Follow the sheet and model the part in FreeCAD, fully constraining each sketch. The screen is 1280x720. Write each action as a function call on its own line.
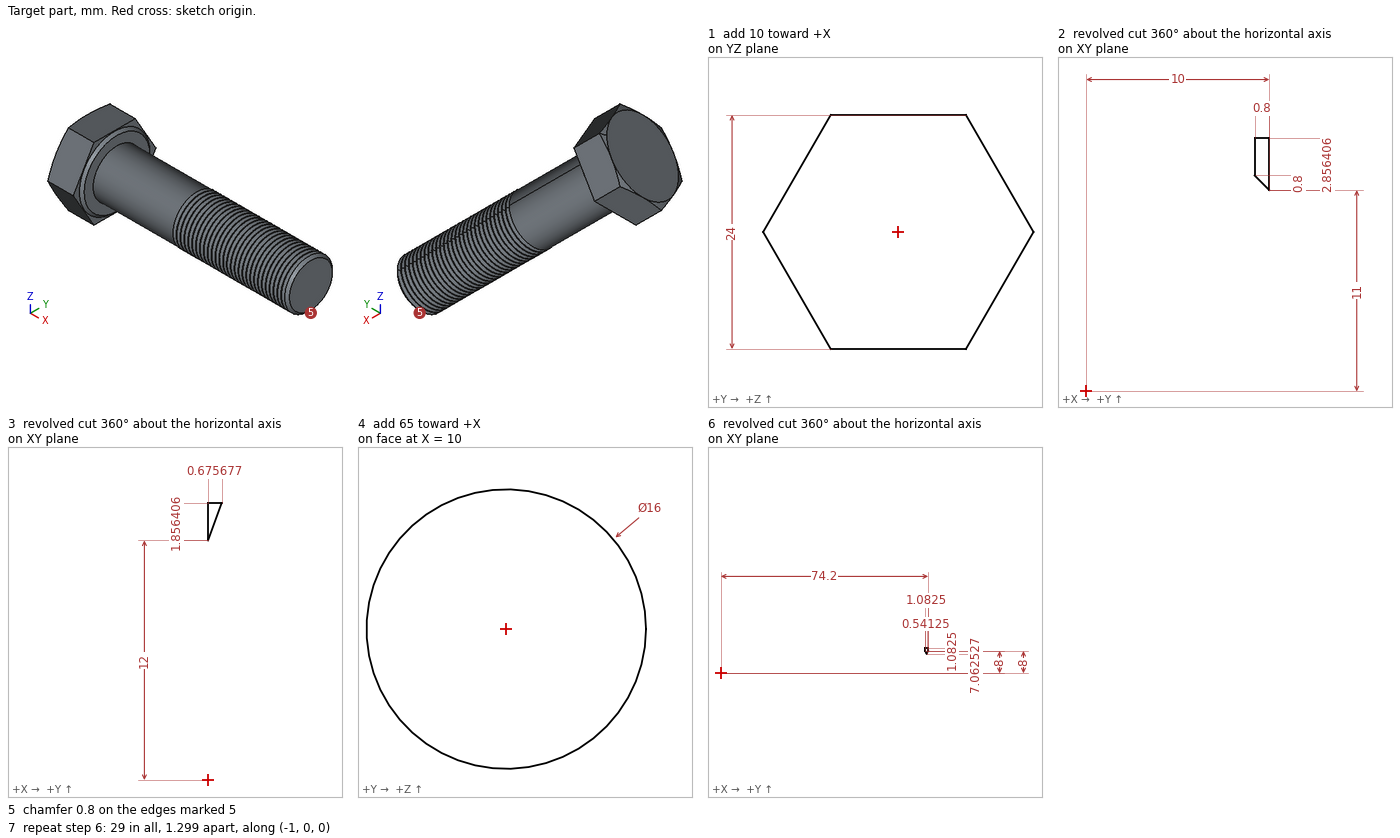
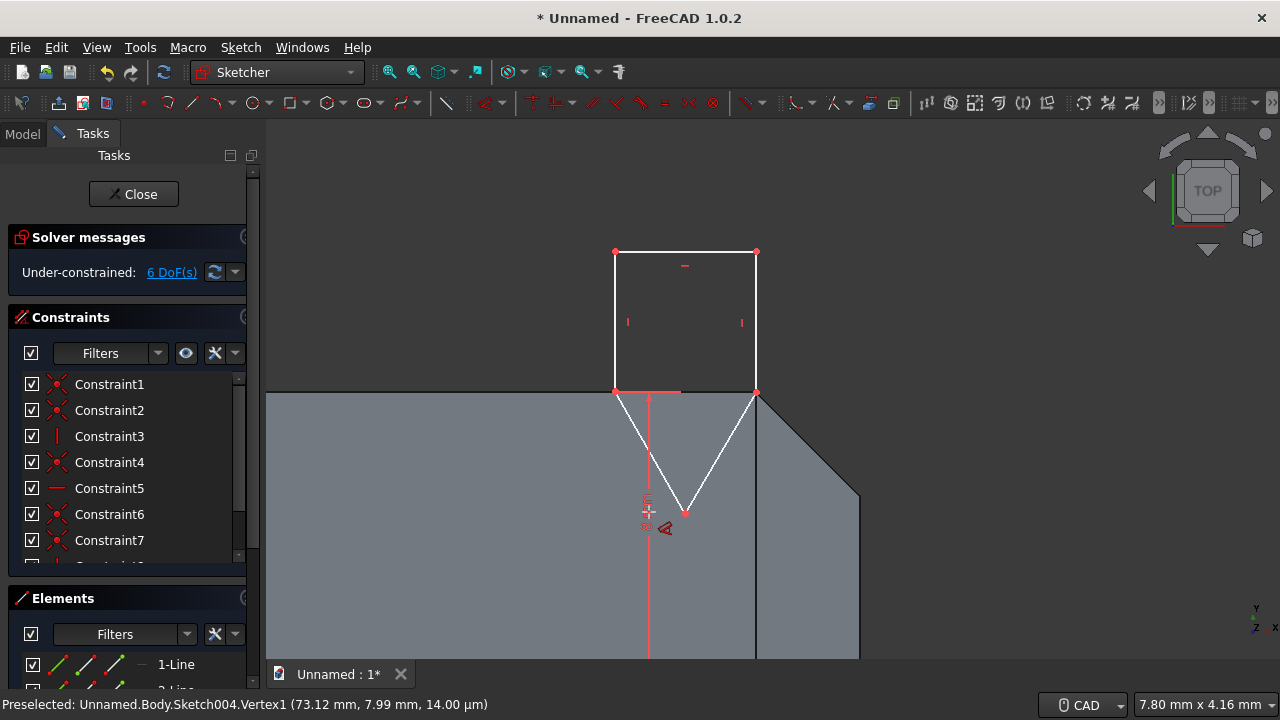
click(756, 393)
click(790, 512)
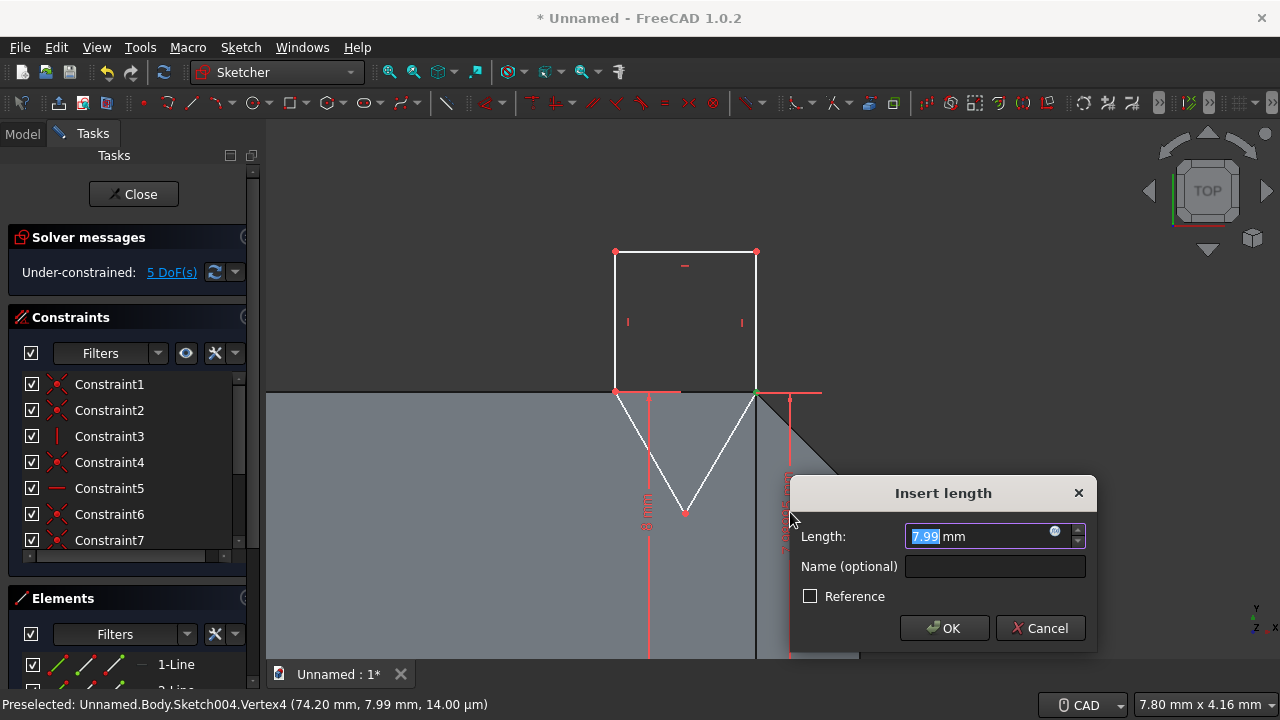
text(8)
key(Return)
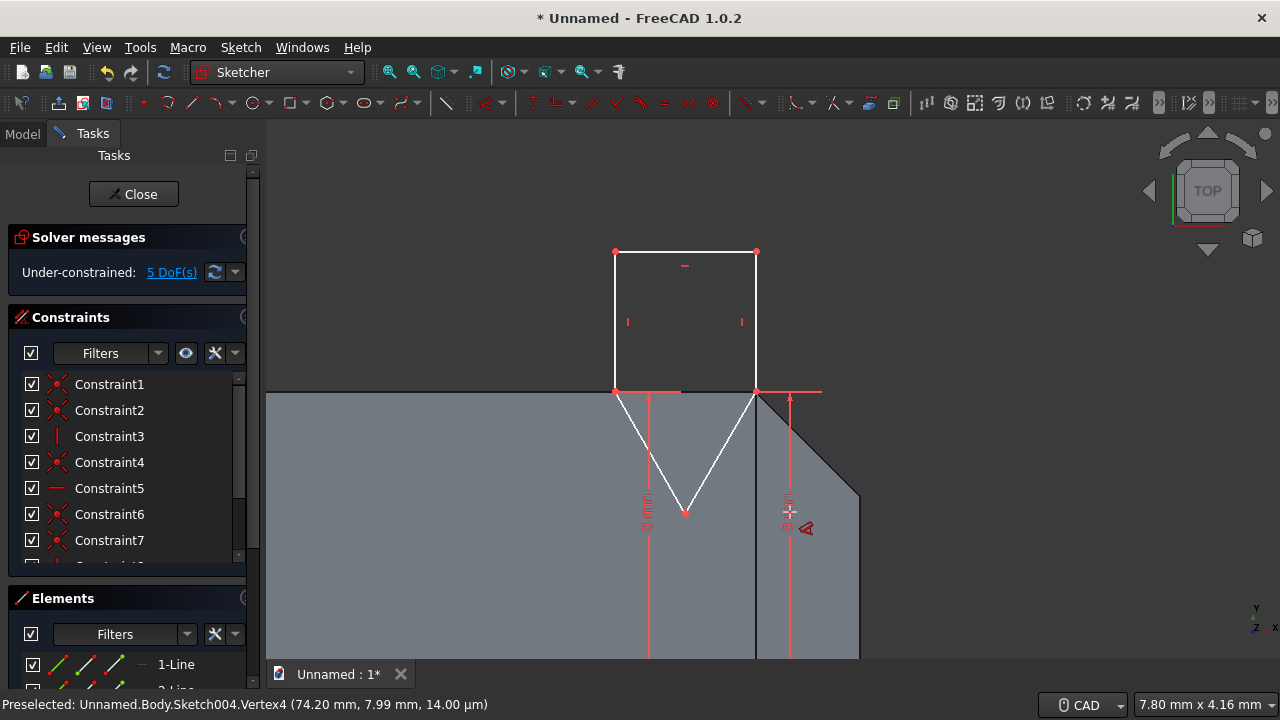
click(756, 392)
click(525, 358)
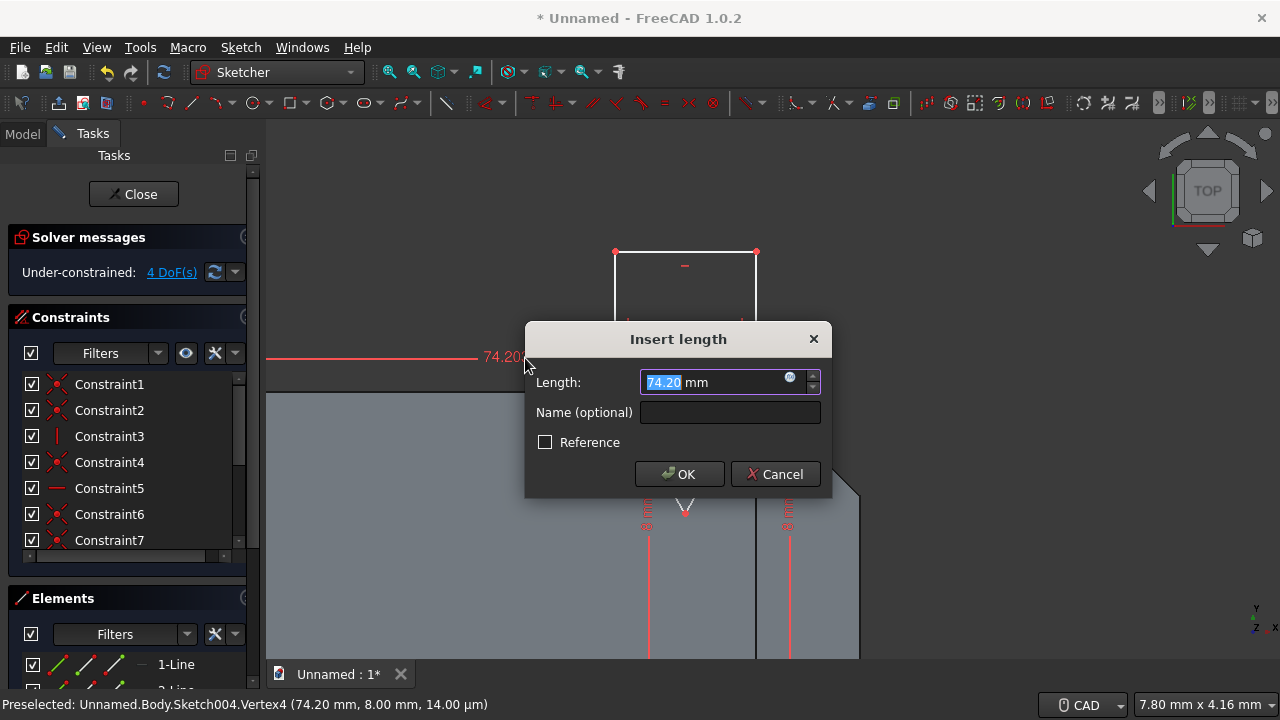
text(74.2)
key(Return)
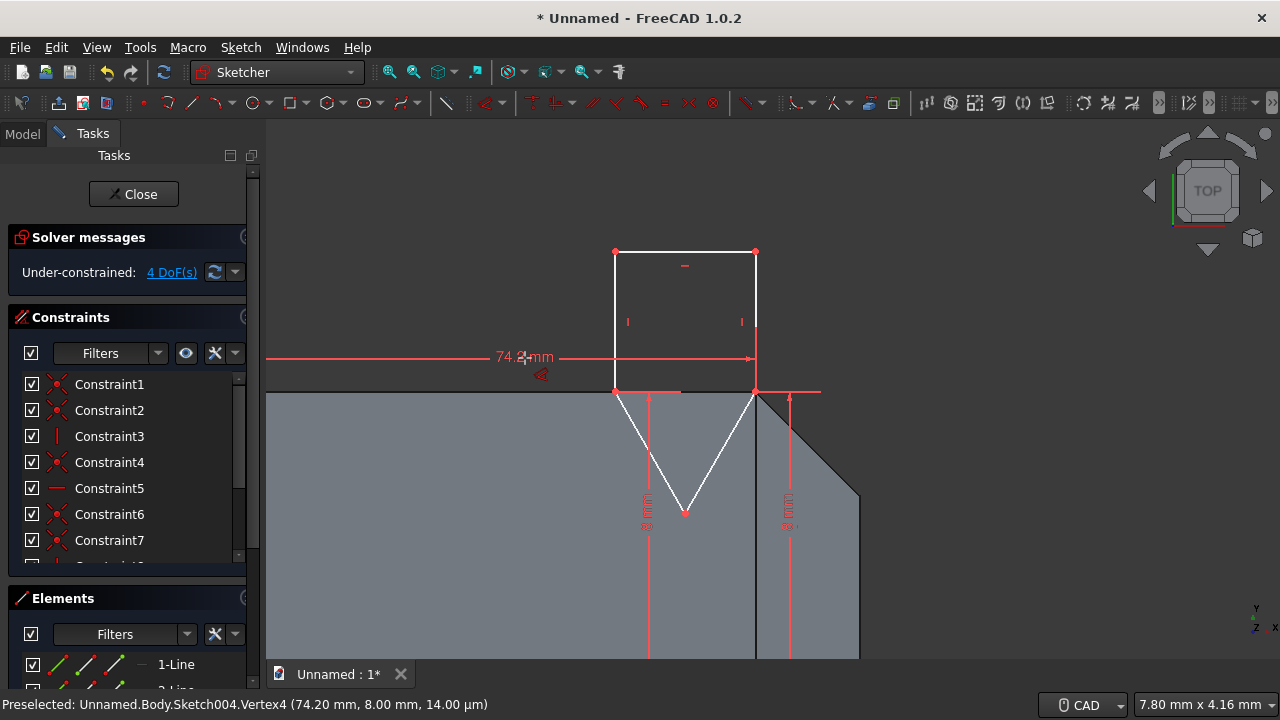
click(756, 350)
click(790, 322)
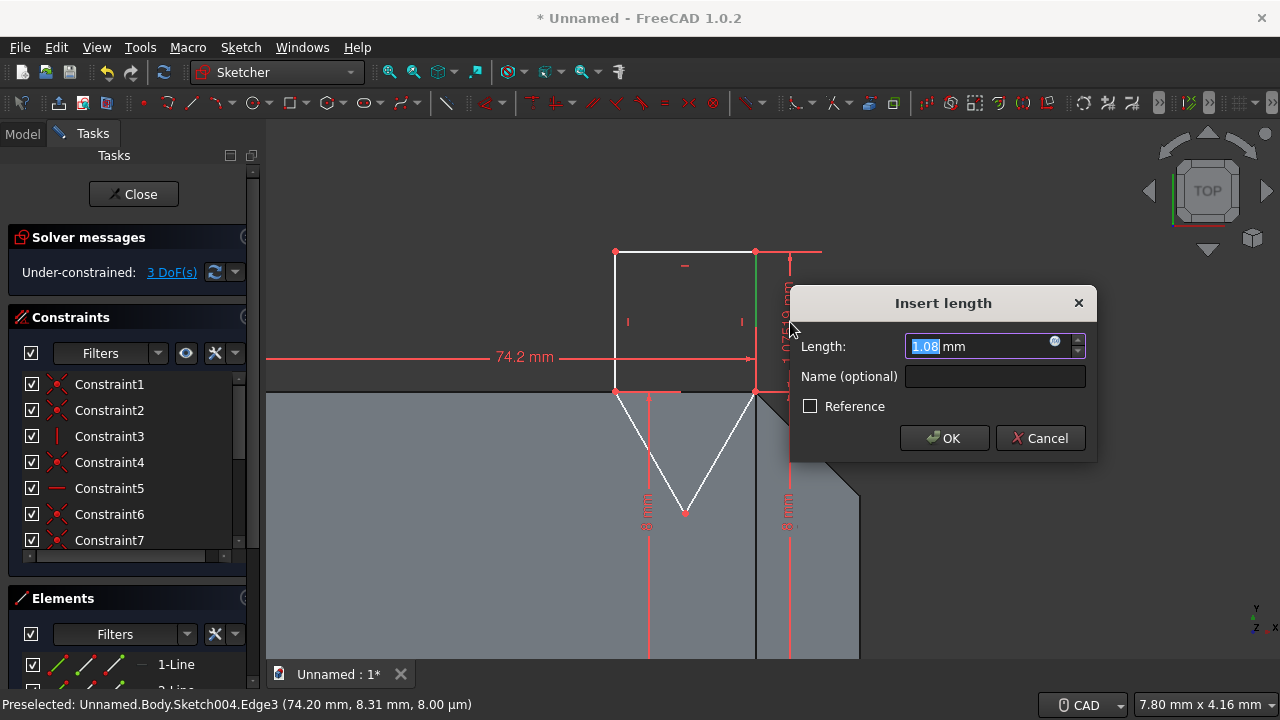
text(1.0825)
key(Return)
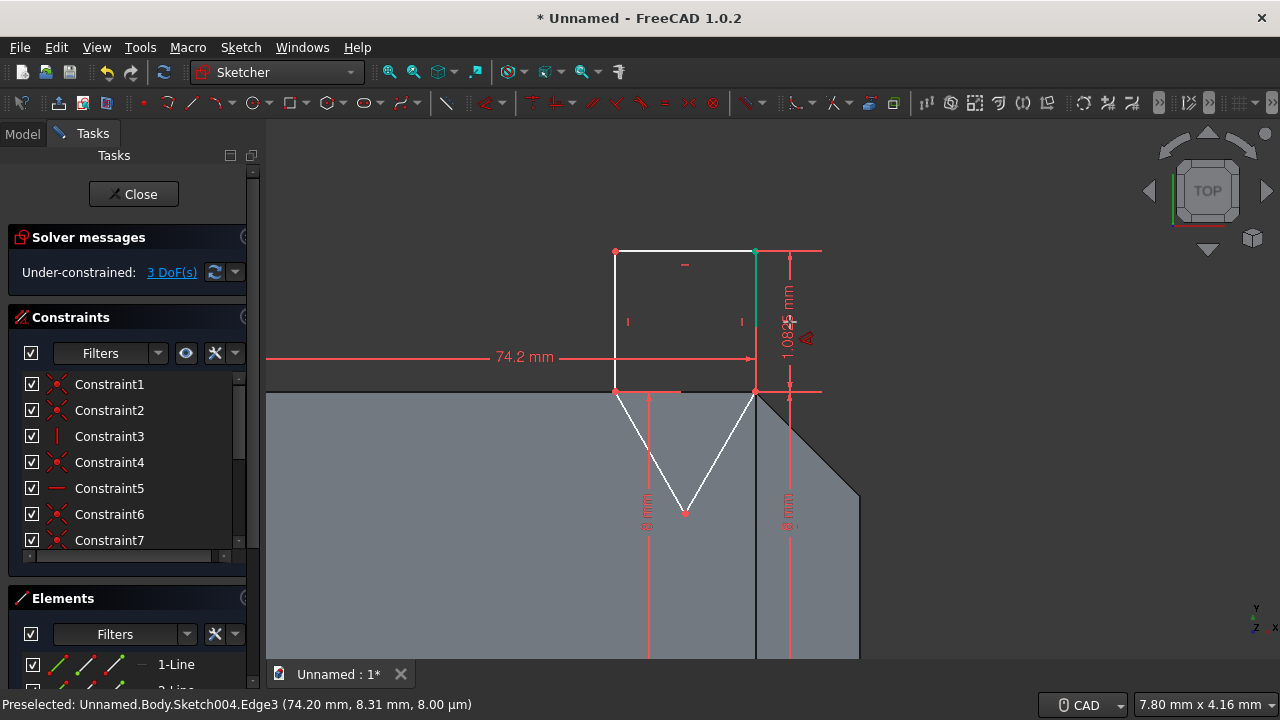
click(713, 251)
click(685, 217)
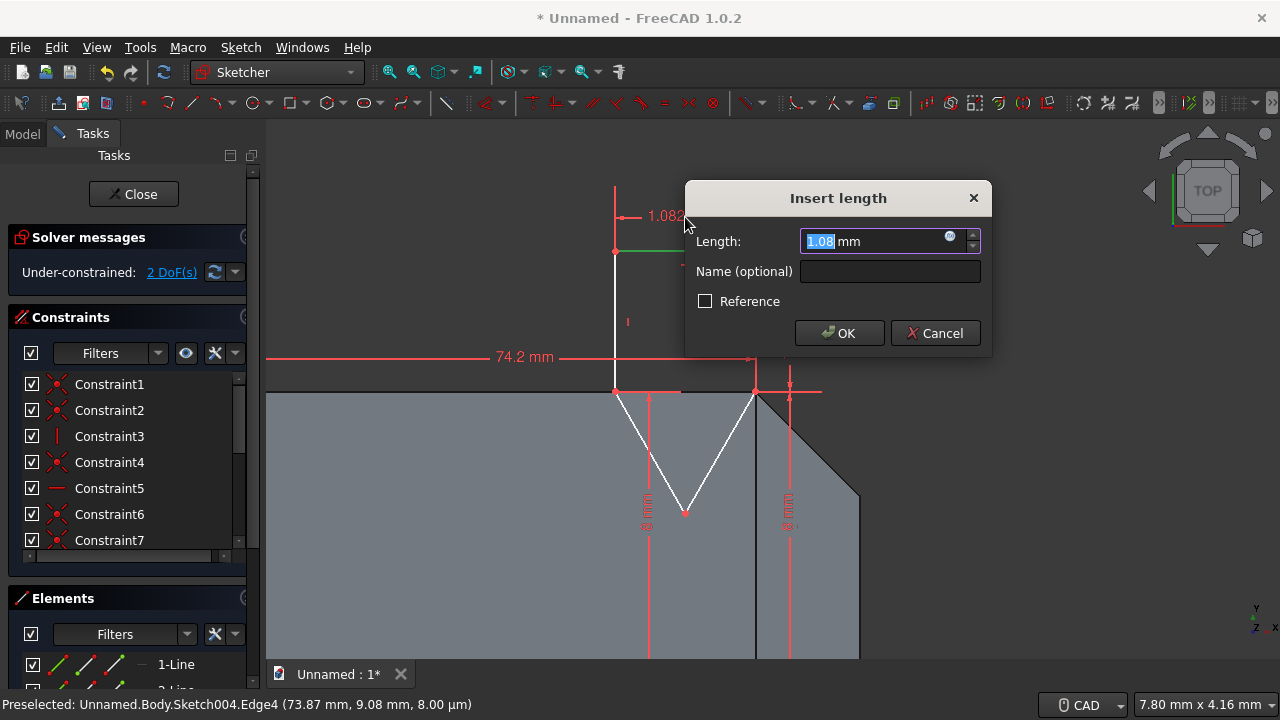
text(1.0825)
key(Return)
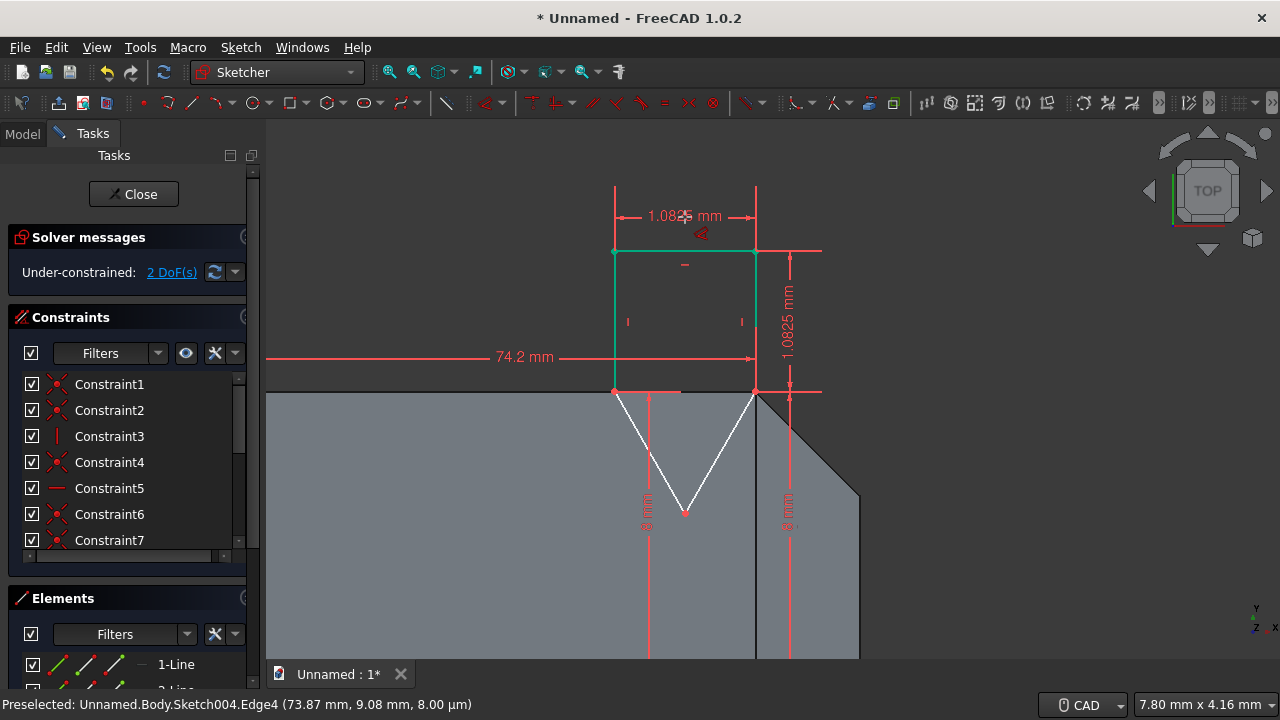
click(636, 428)
click(650, 548)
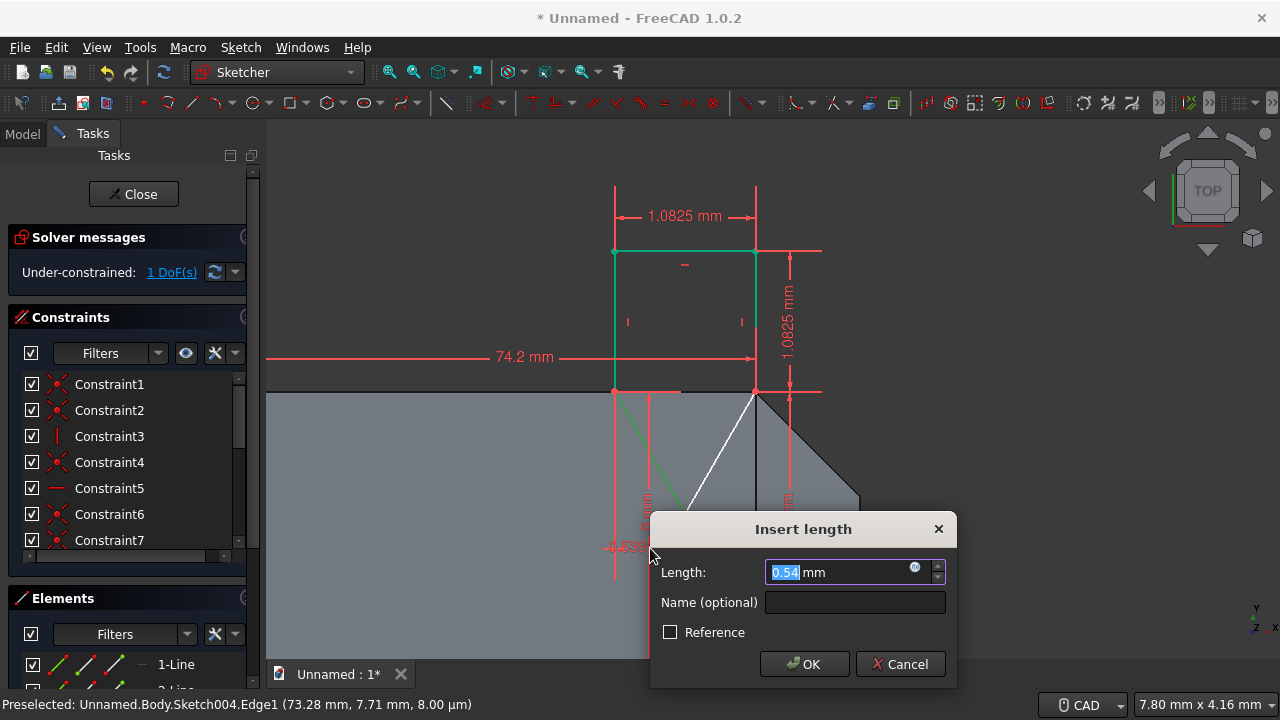
text(0.54125)
key(Return)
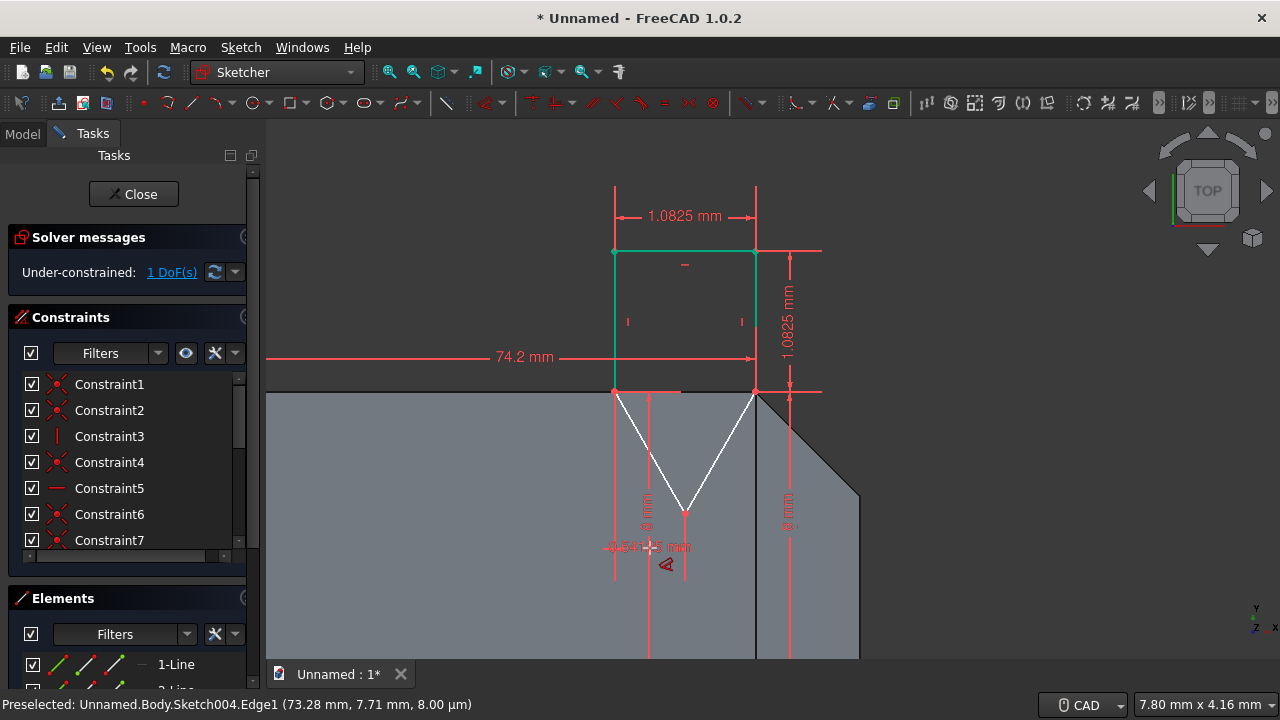
click(685, 514)
click(719, 573)